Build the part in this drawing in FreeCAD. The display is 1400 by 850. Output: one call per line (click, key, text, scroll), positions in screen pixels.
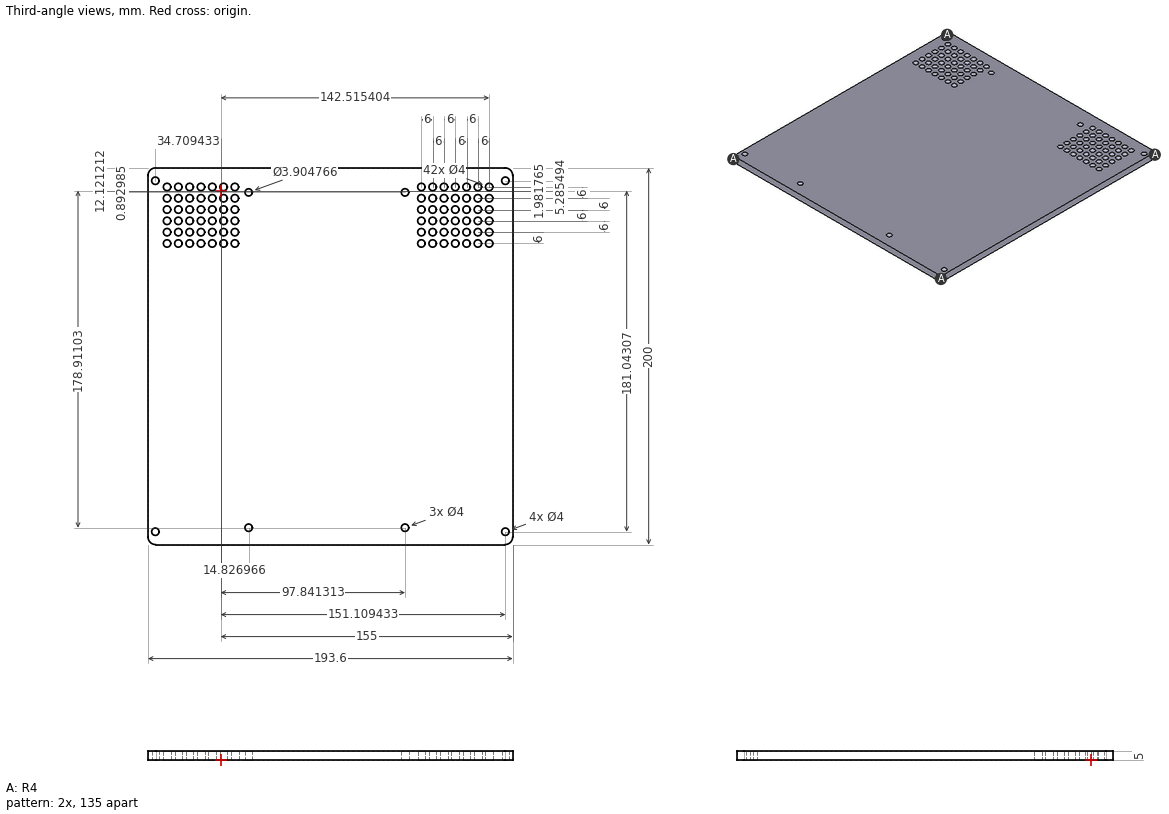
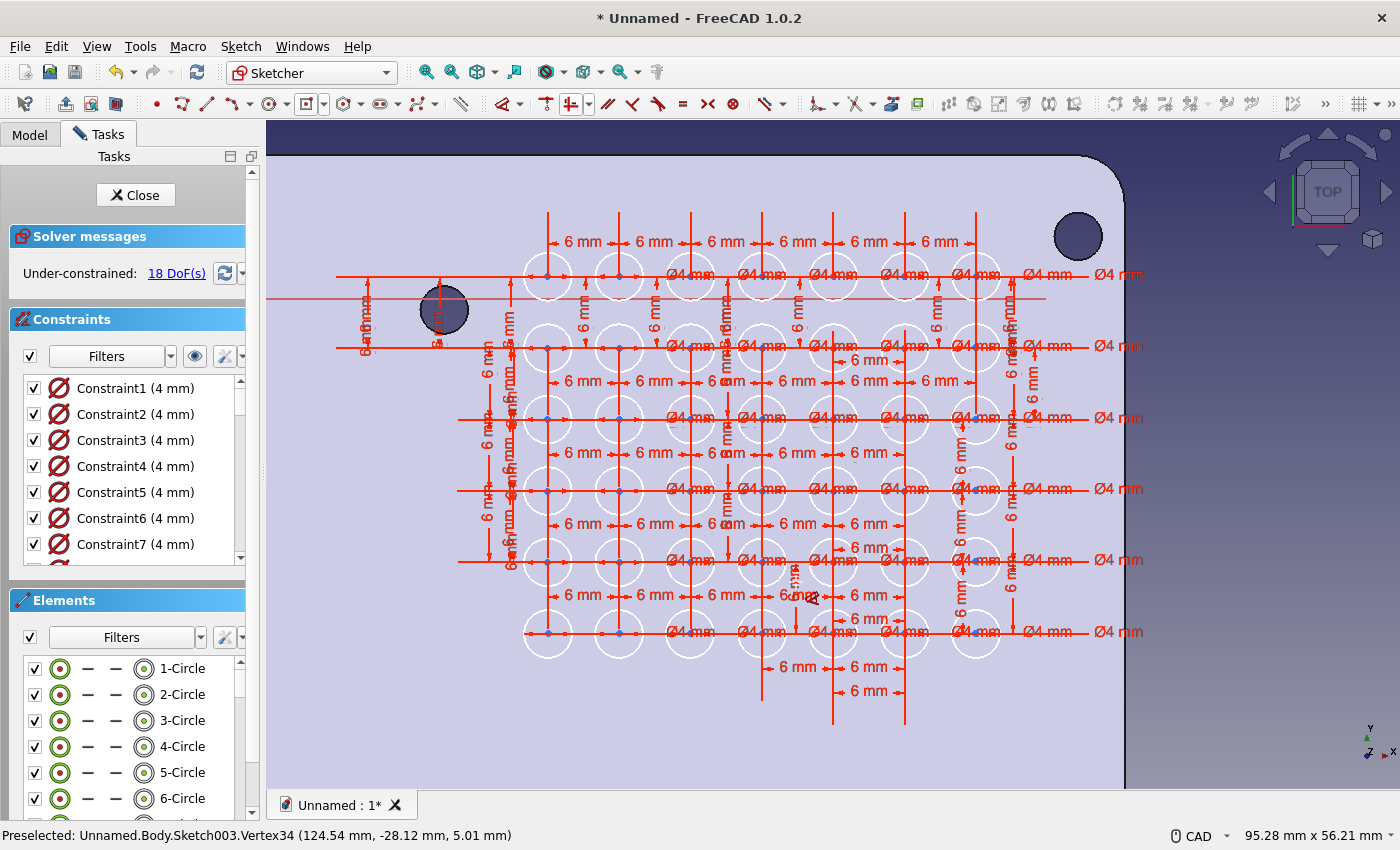
click(762, 634)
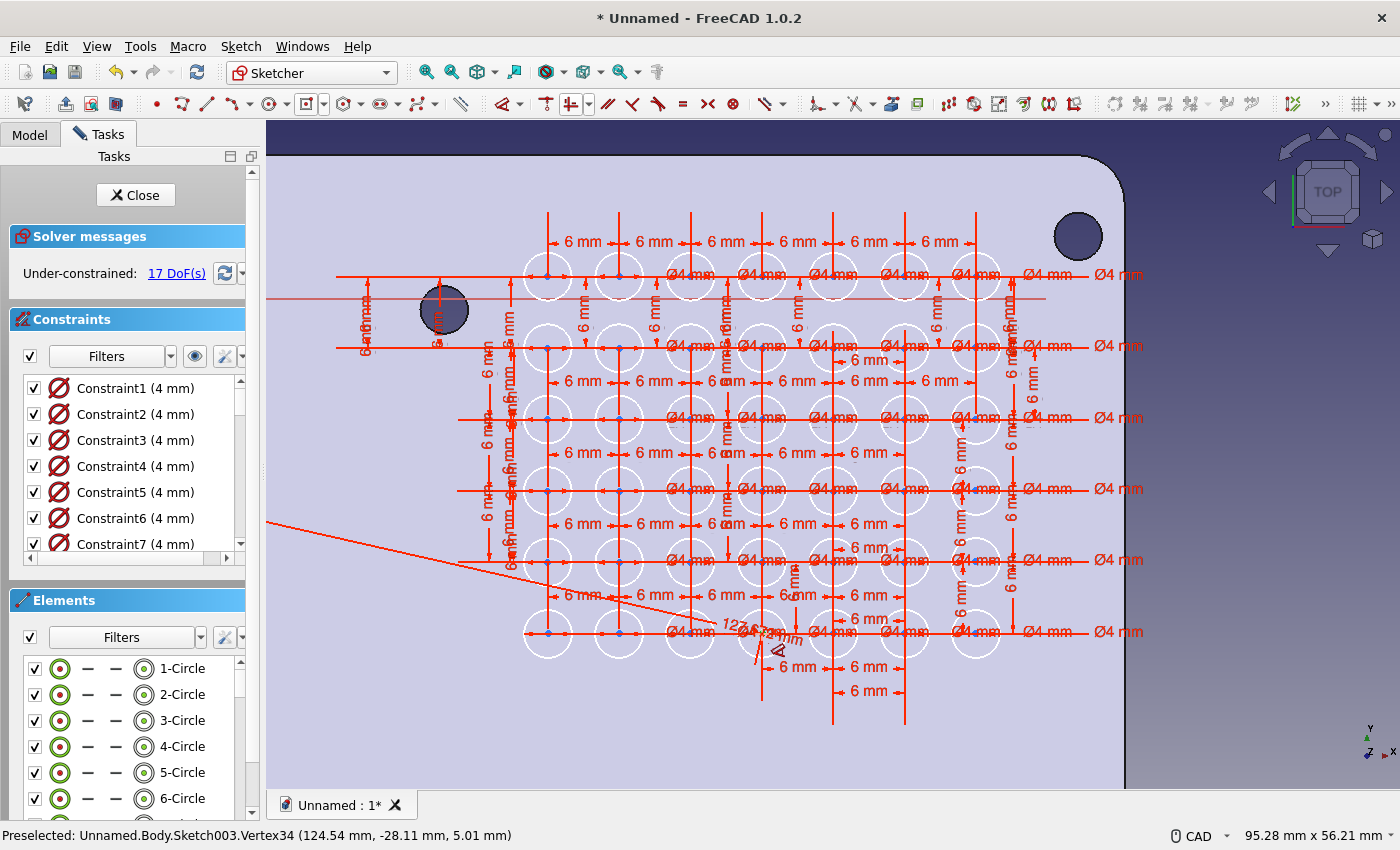
click(690, 634)
click(726, 668)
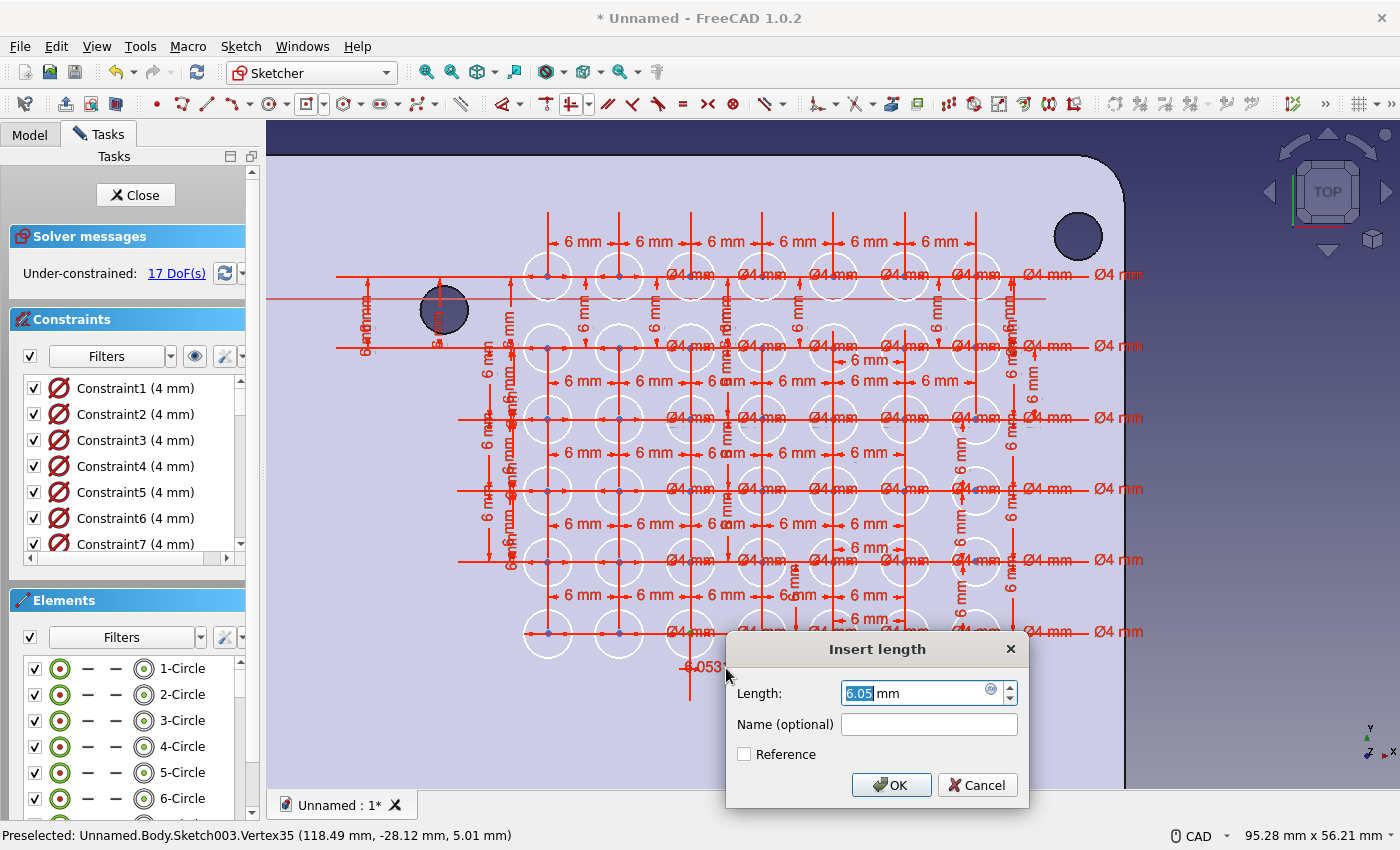
text(6)
key(Return)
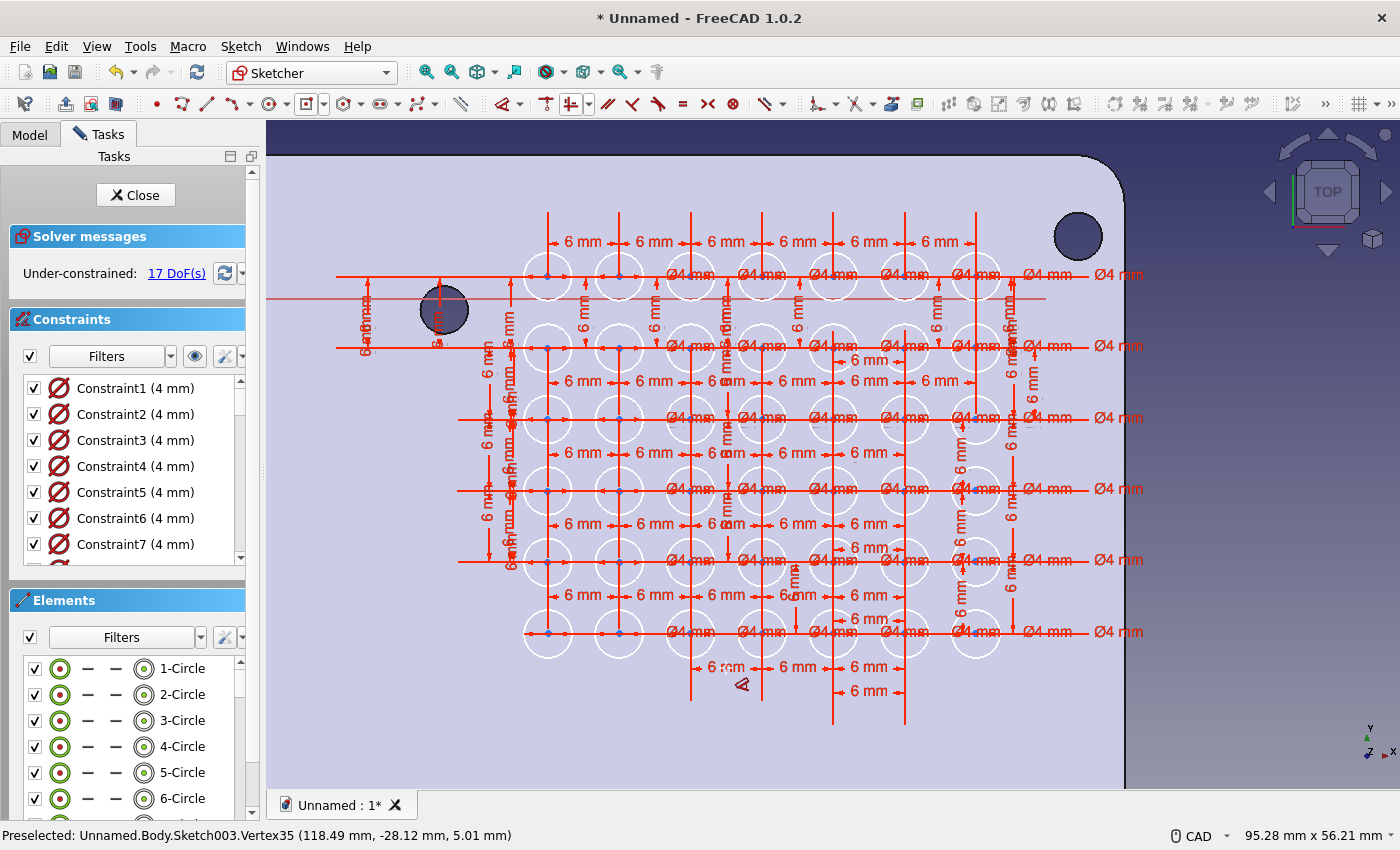
click(691, 562)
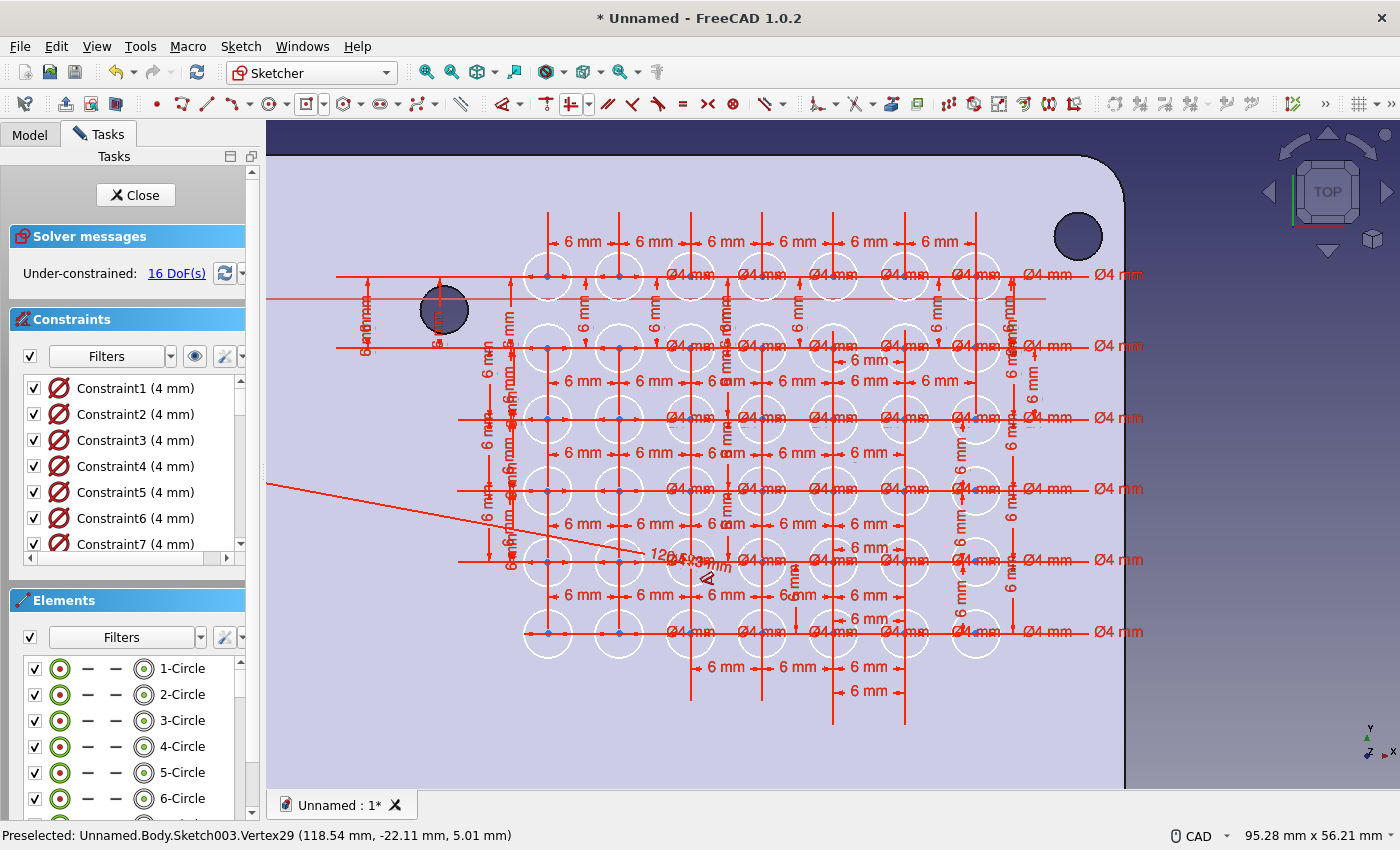
click(691, 634)
click(511, 598)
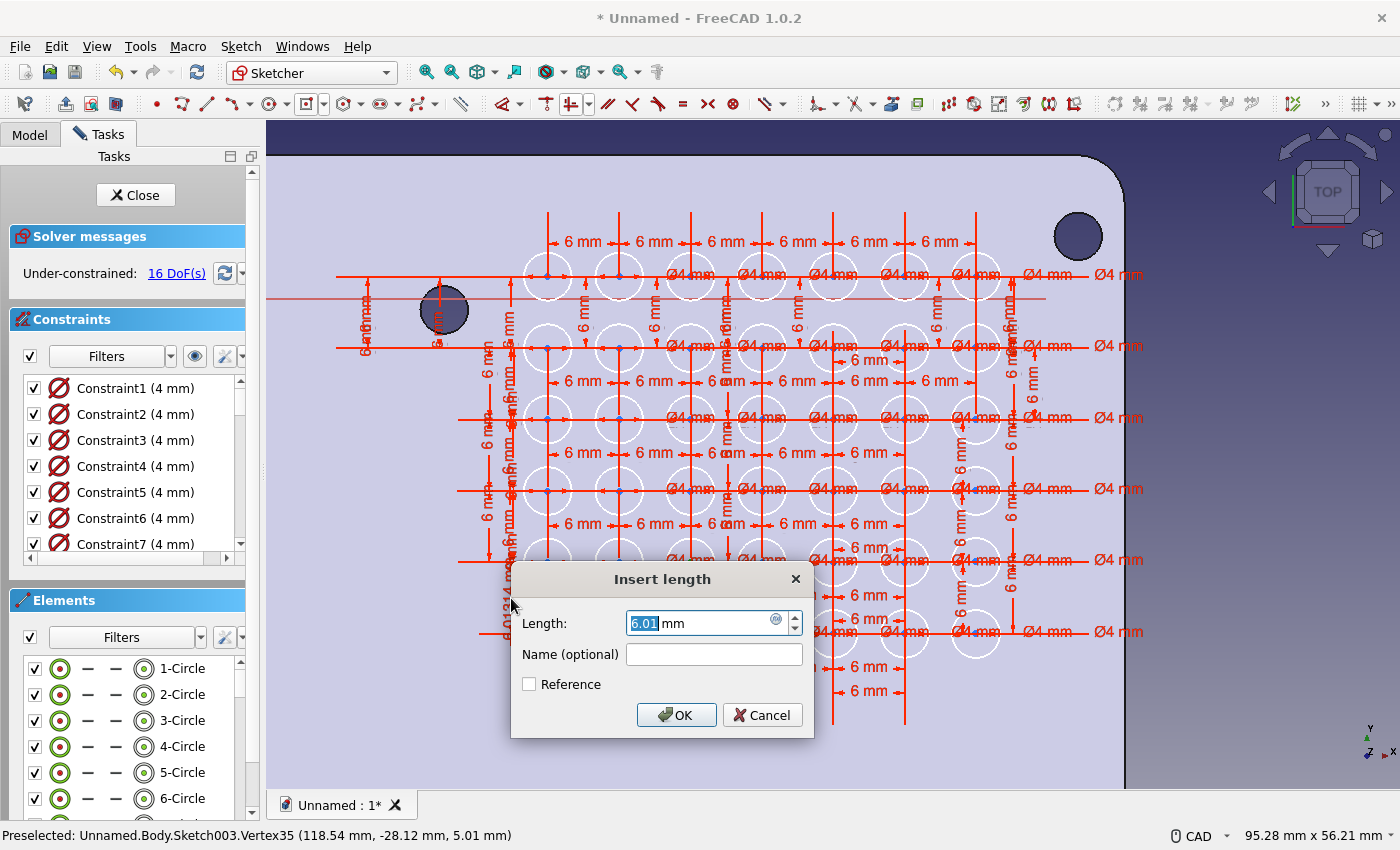
text(6)
key(Return)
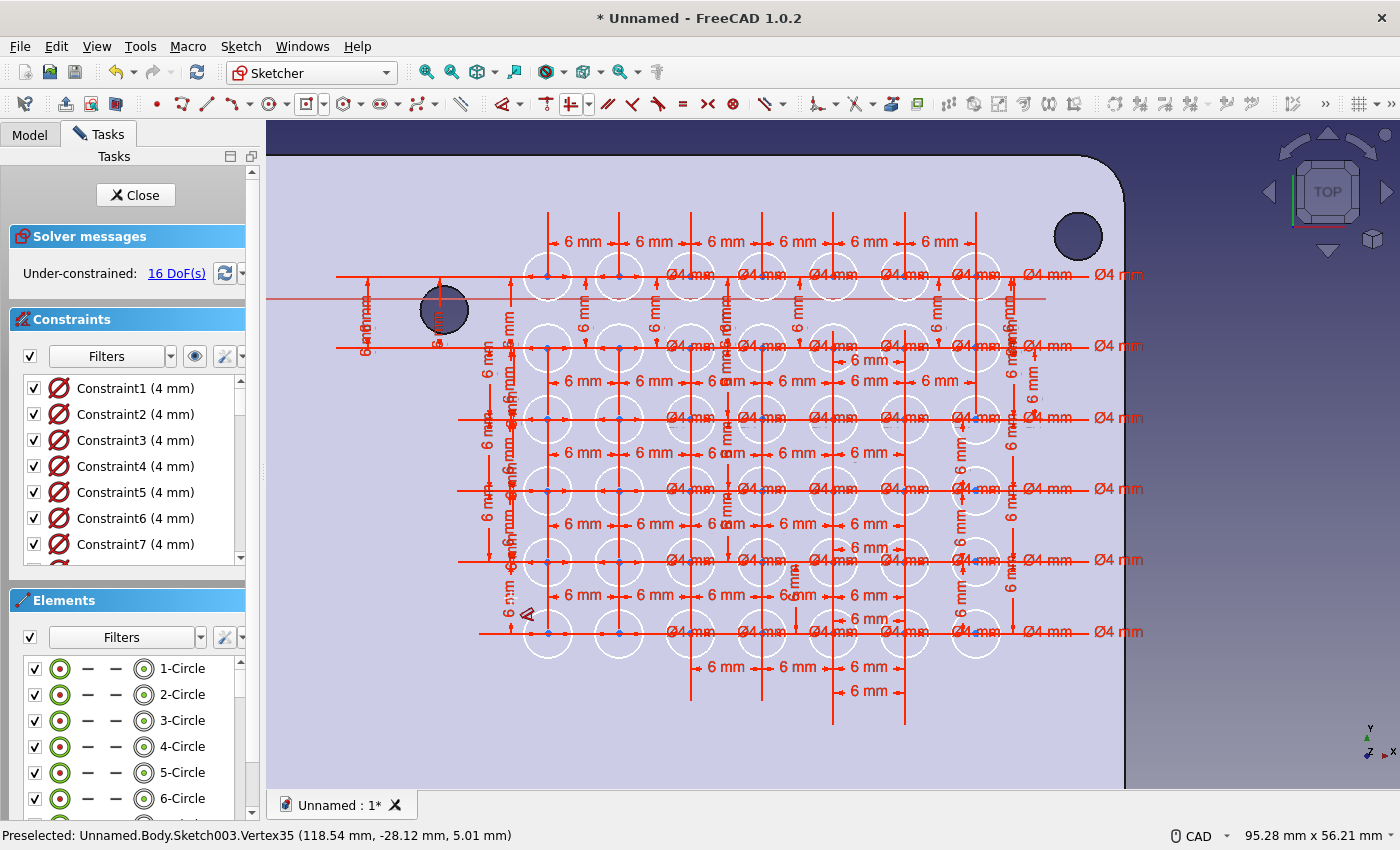
click(691, 634)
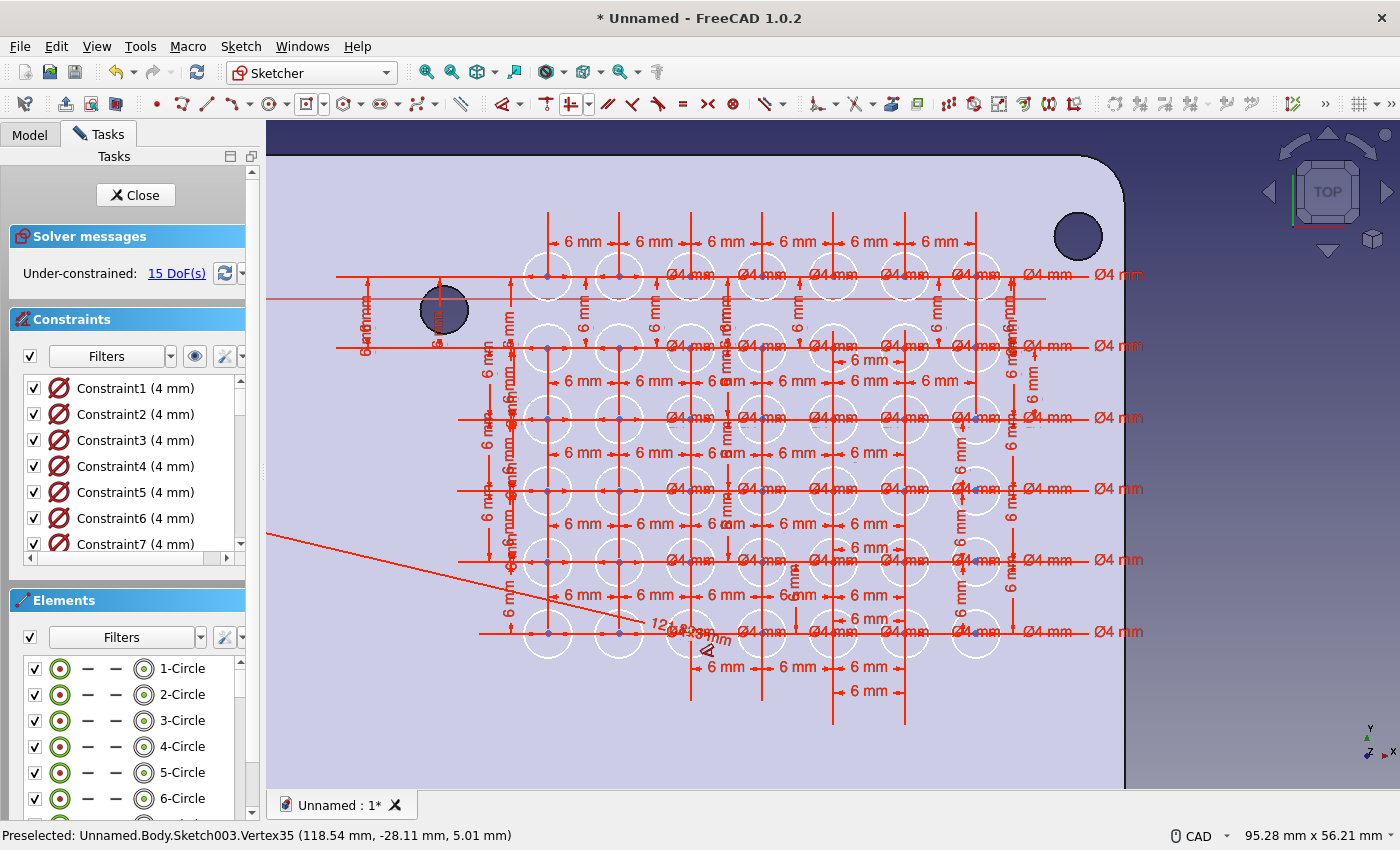
click(619, 634)
click(655, 668)